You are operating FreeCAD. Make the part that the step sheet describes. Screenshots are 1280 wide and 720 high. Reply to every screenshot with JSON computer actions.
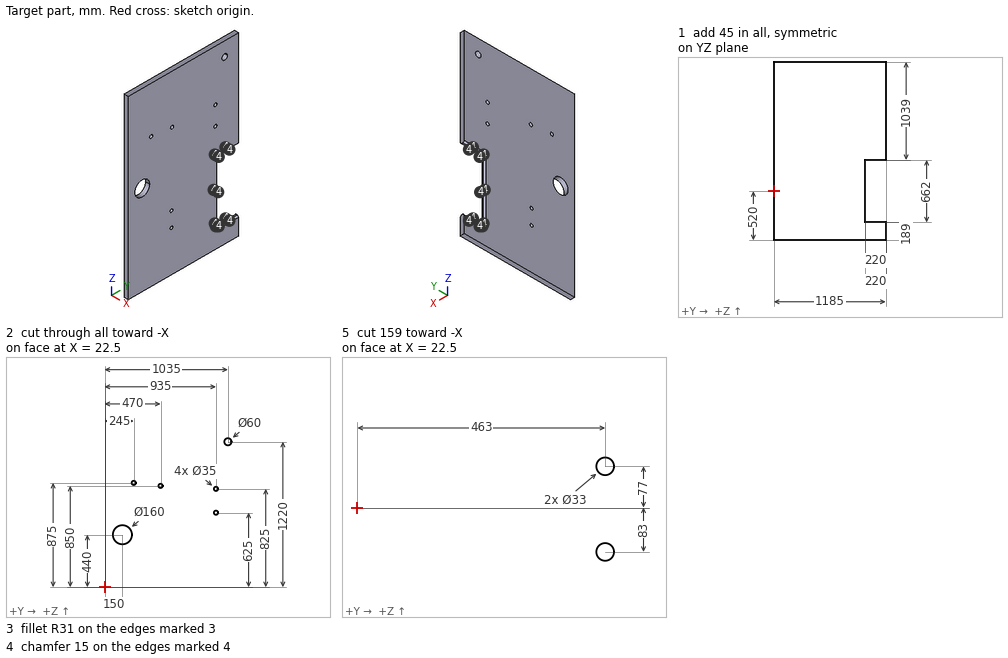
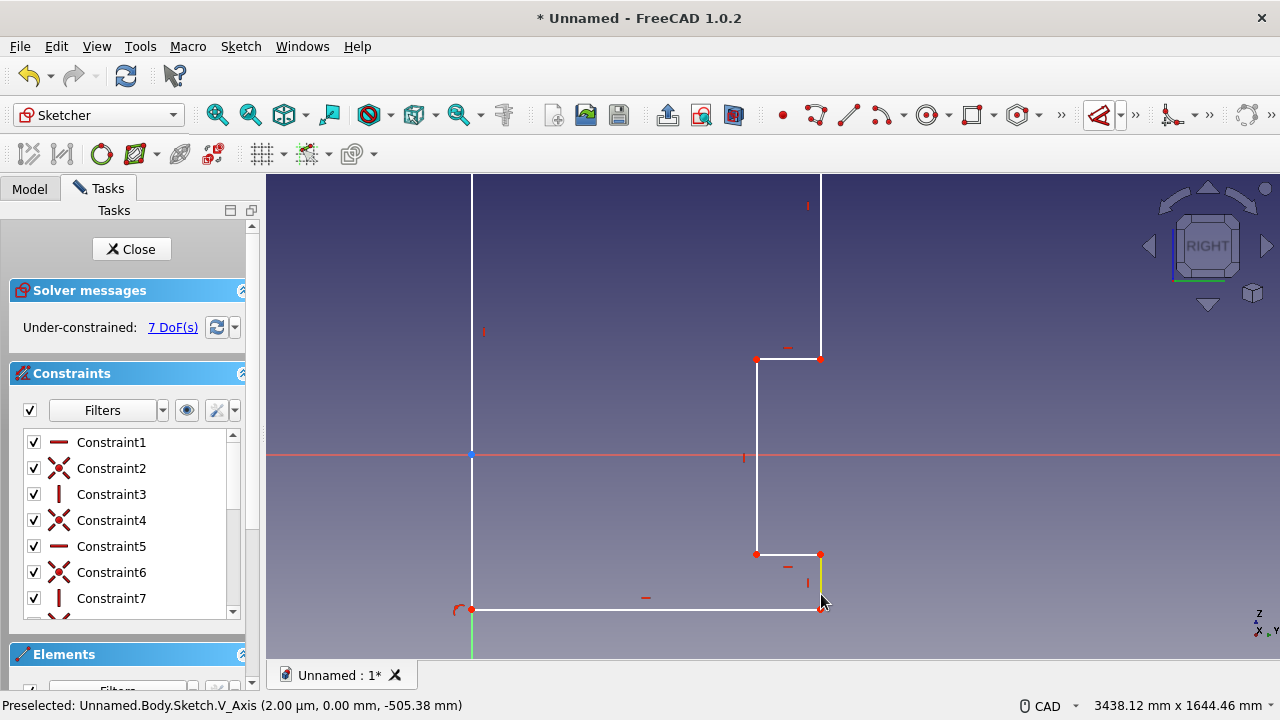
{"action": "left_click", "coordinate": [821, 593]}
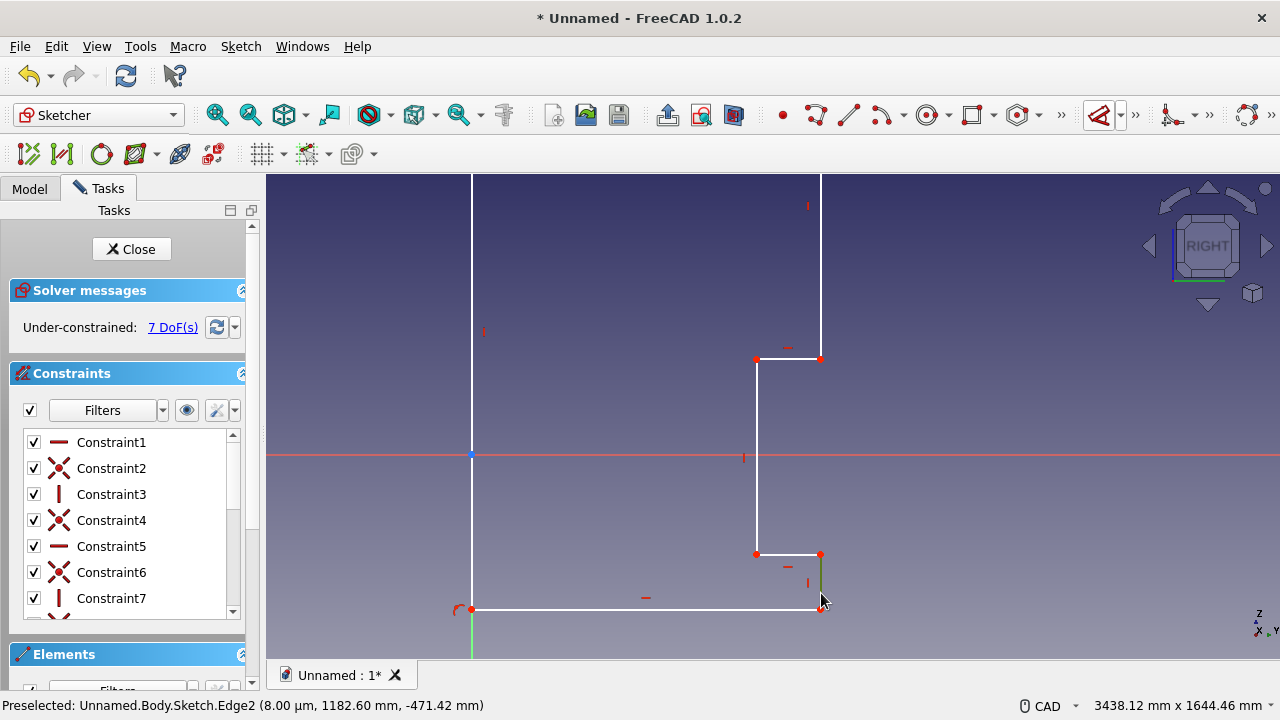
{"action": "left_click", "coordinate": [1120, 116]}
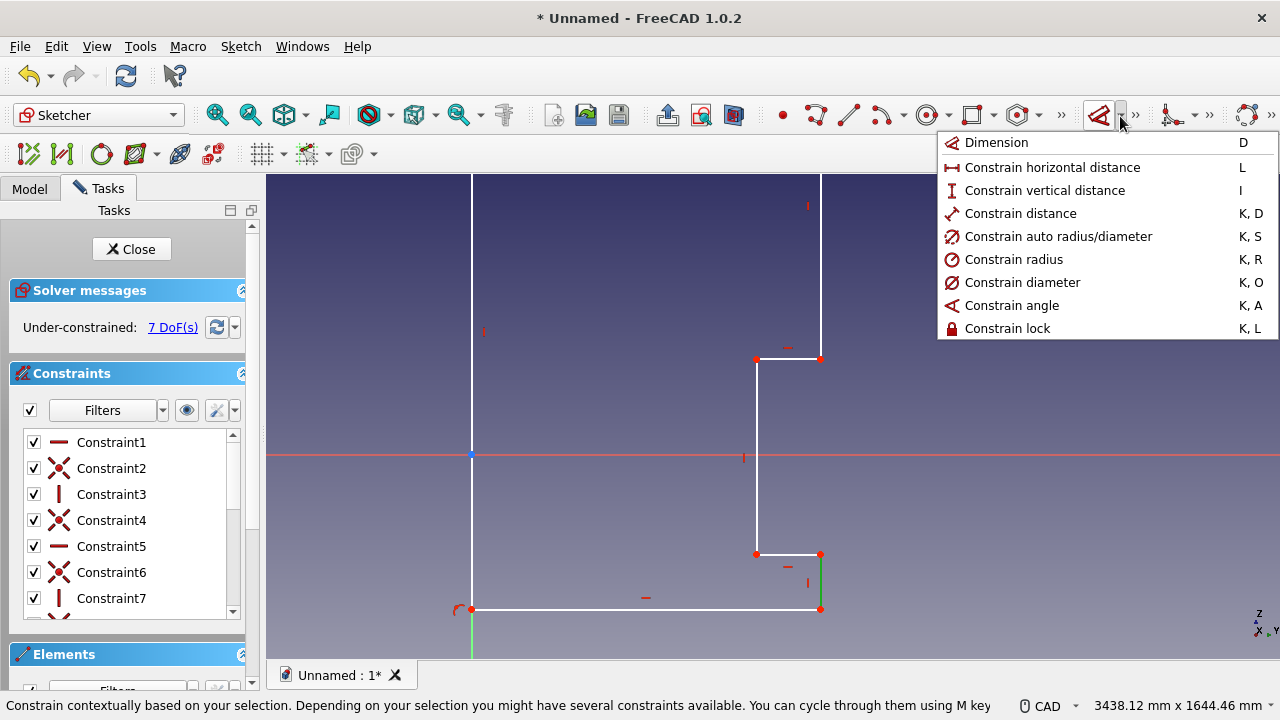
{"action": "left_click", "coordinate": [1108, 190]}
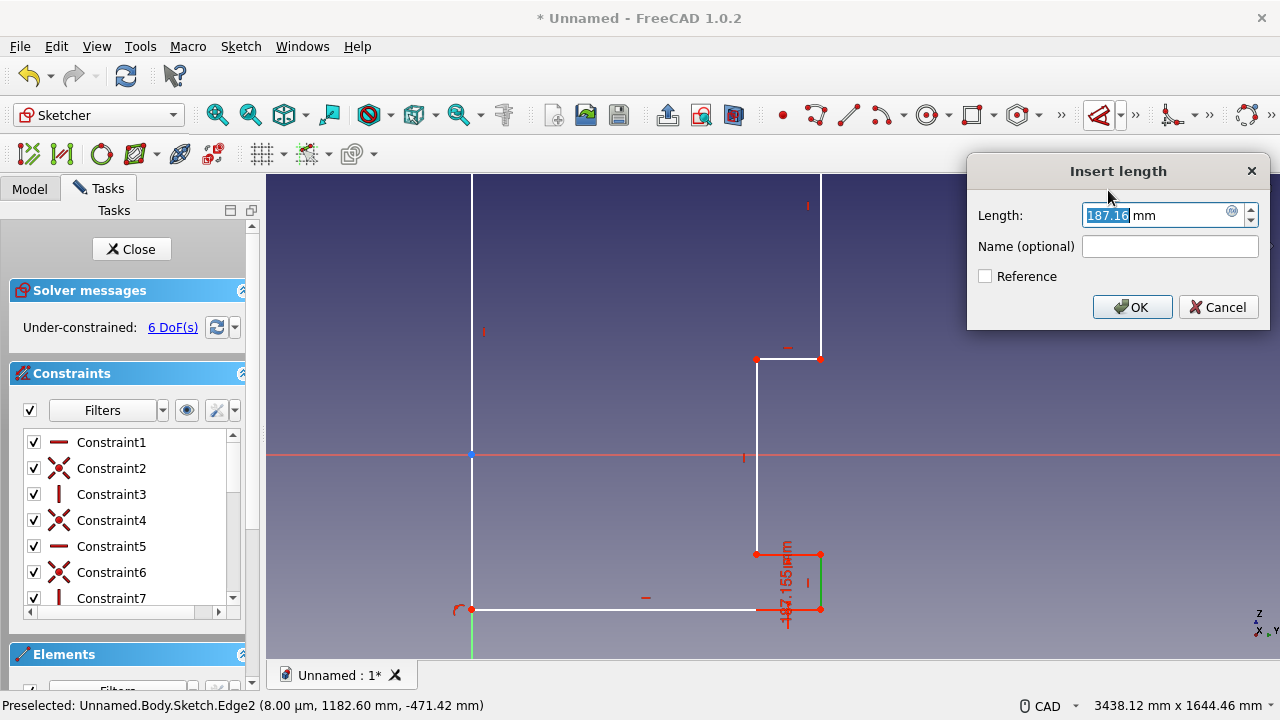
{"action": "type", "text": "189"}
{"action": "key", "text": "Return"}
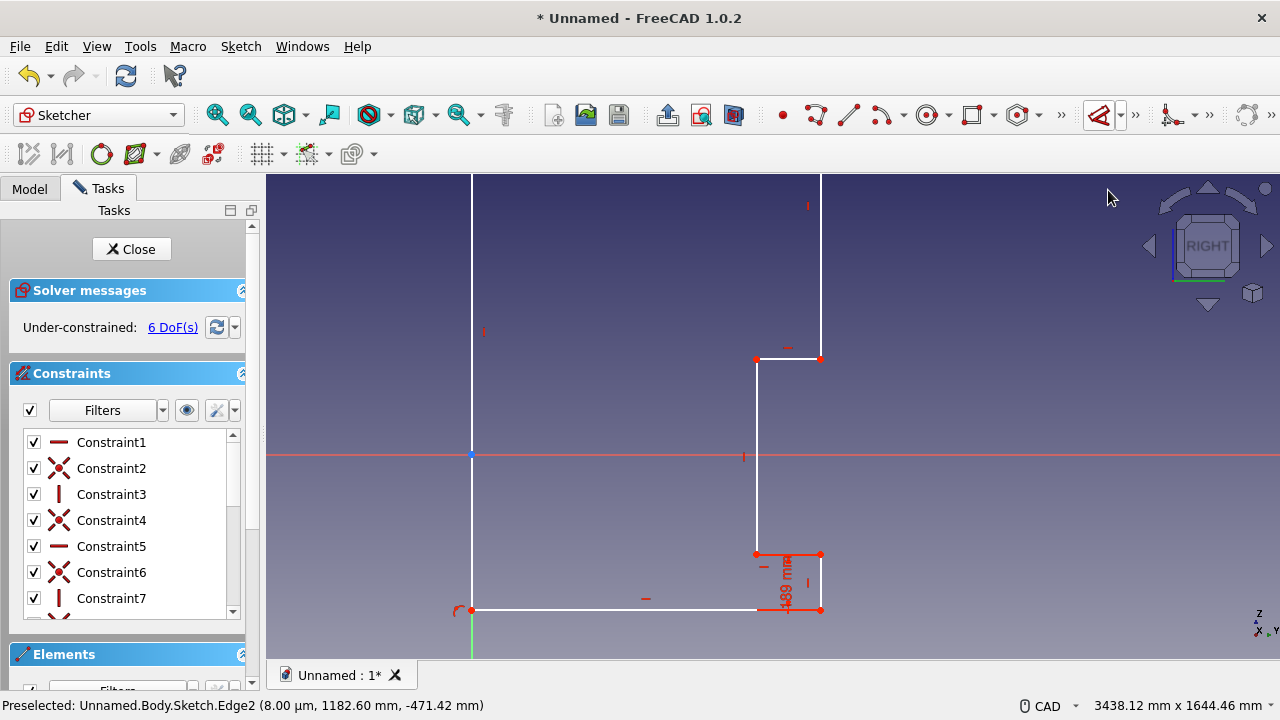
{"action": "left_click", "coordinate": [801, 555]}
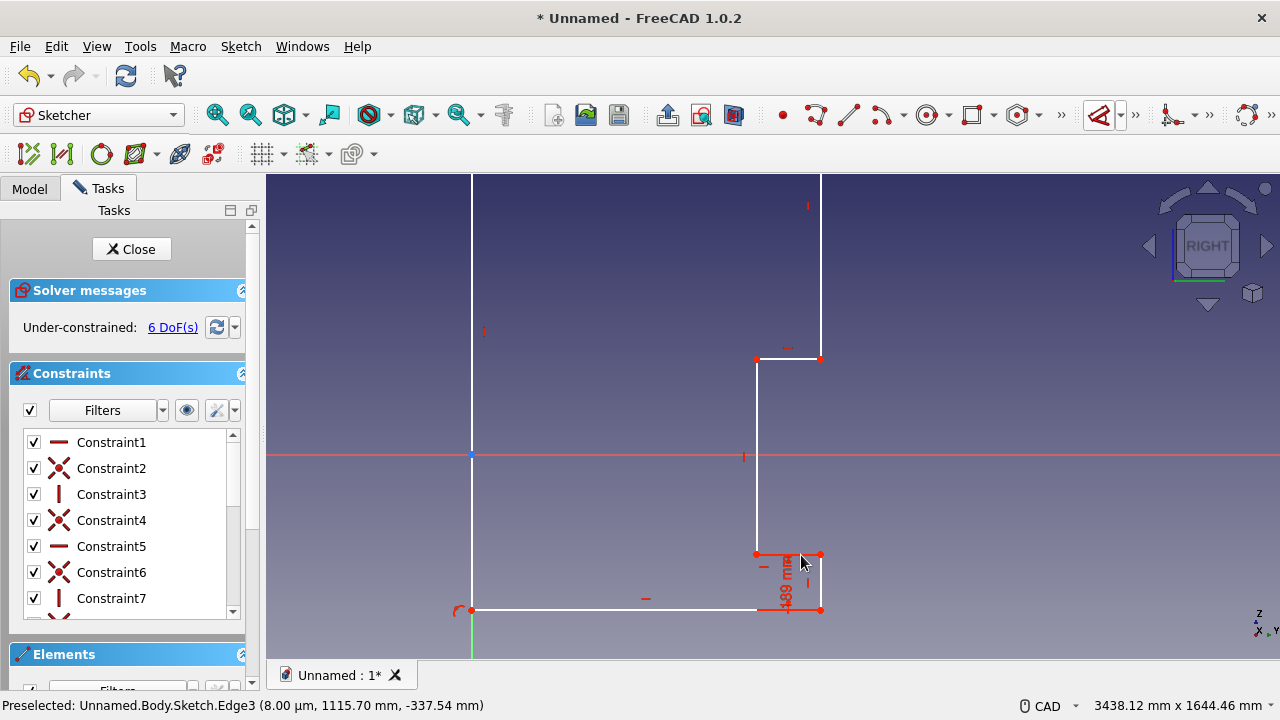
{"action": "left_click", "coordinate": [1120, 116]}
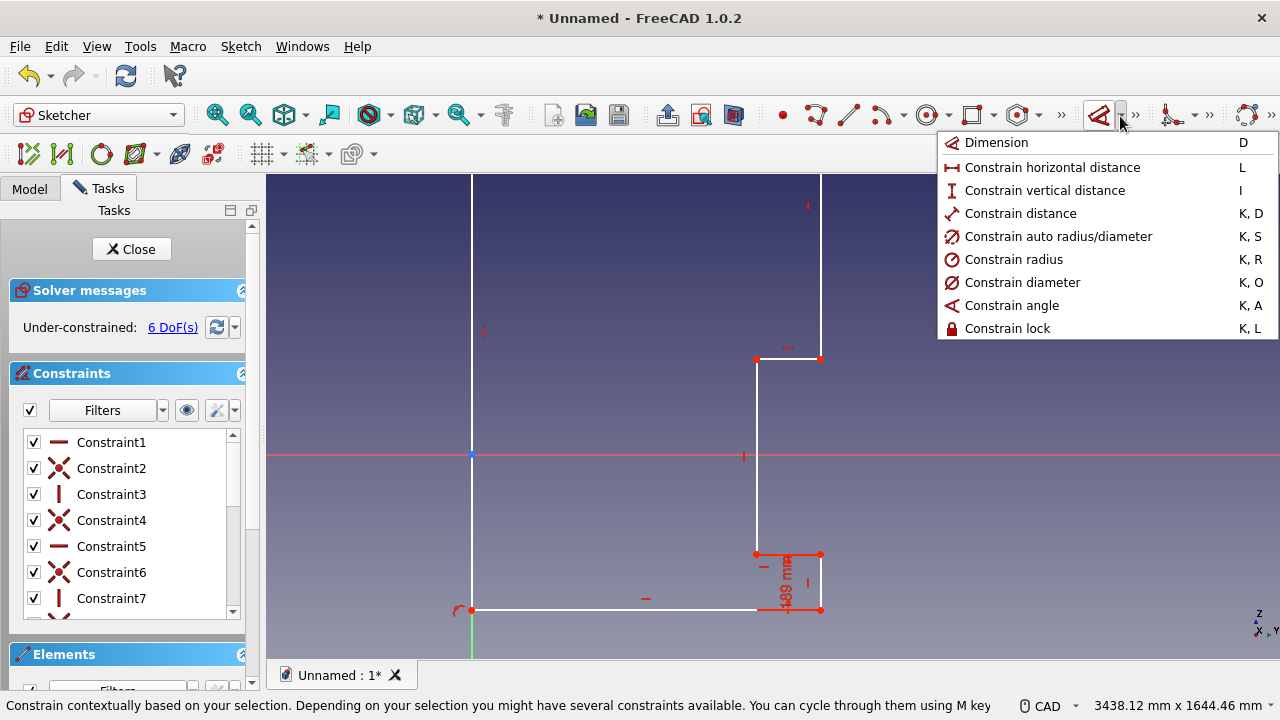
{"action": "left_click", "coordinate": [1108, 168]}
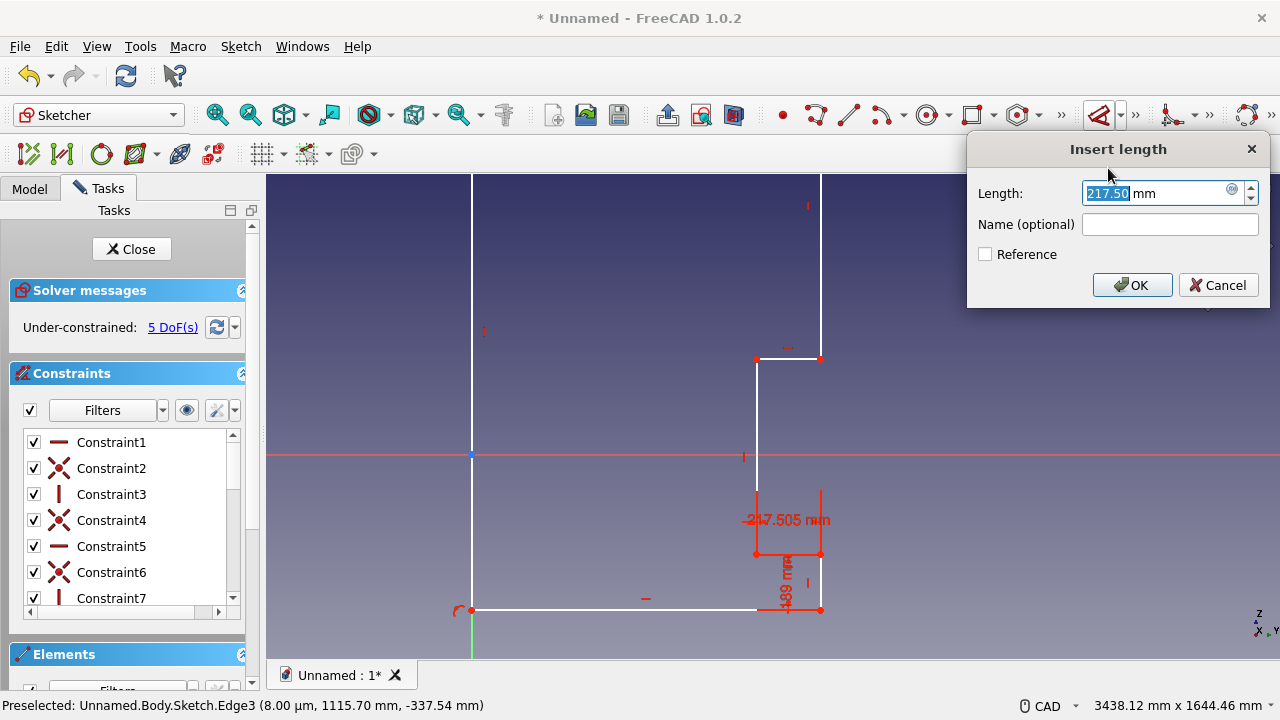
{"action": "type", "text": "220"}
{"action": "key", "text": "Return"}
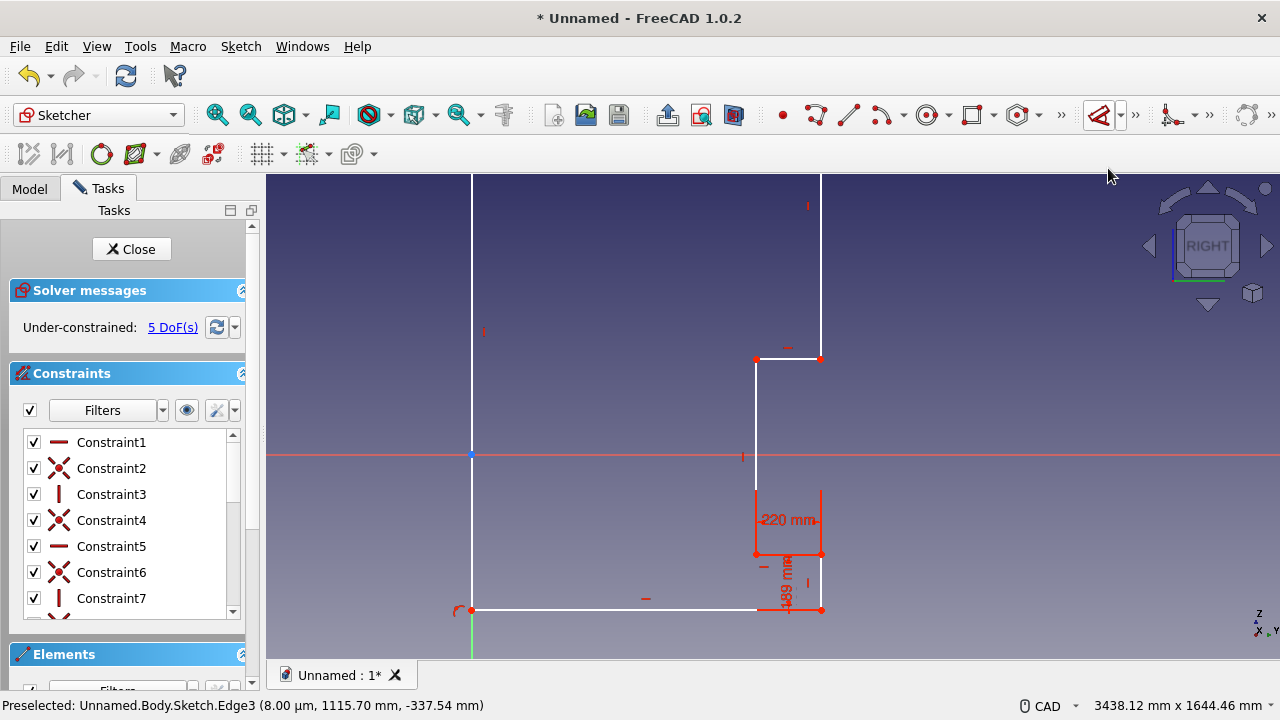
{"action": "left_click", "coordinate": [756, 496]}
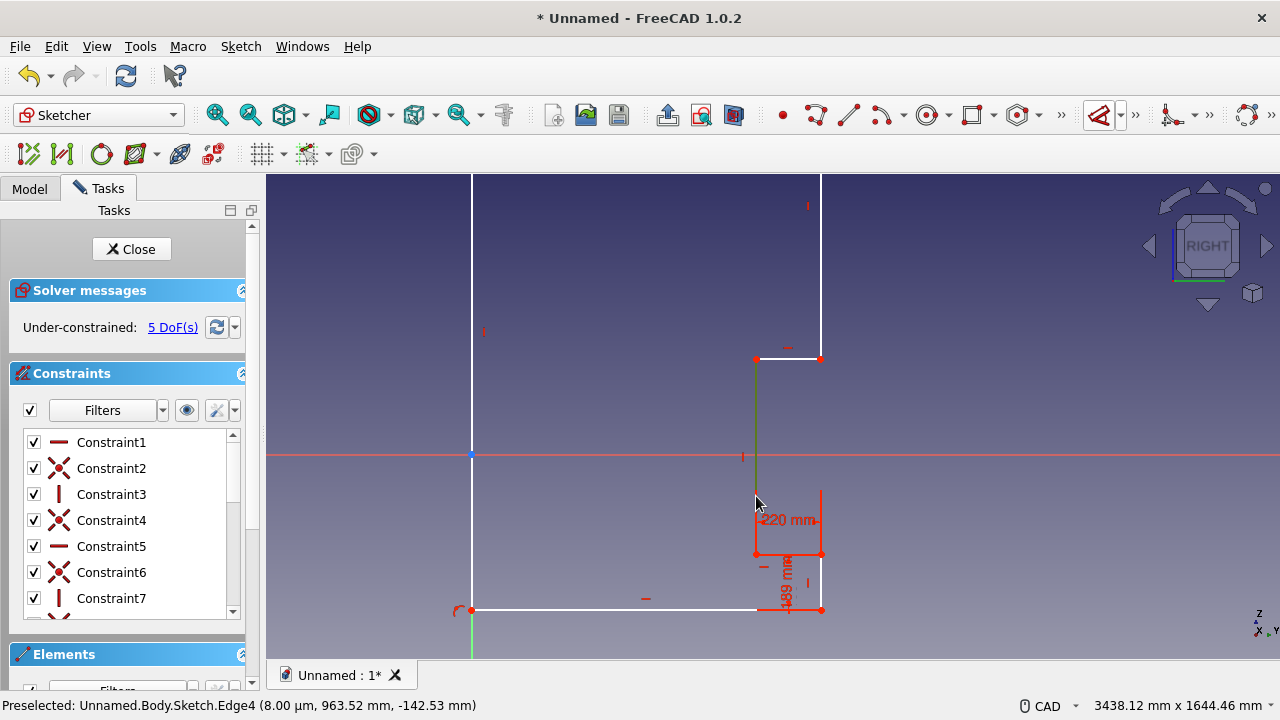
{"action": "left_click", "coordinate": [1120, 116]}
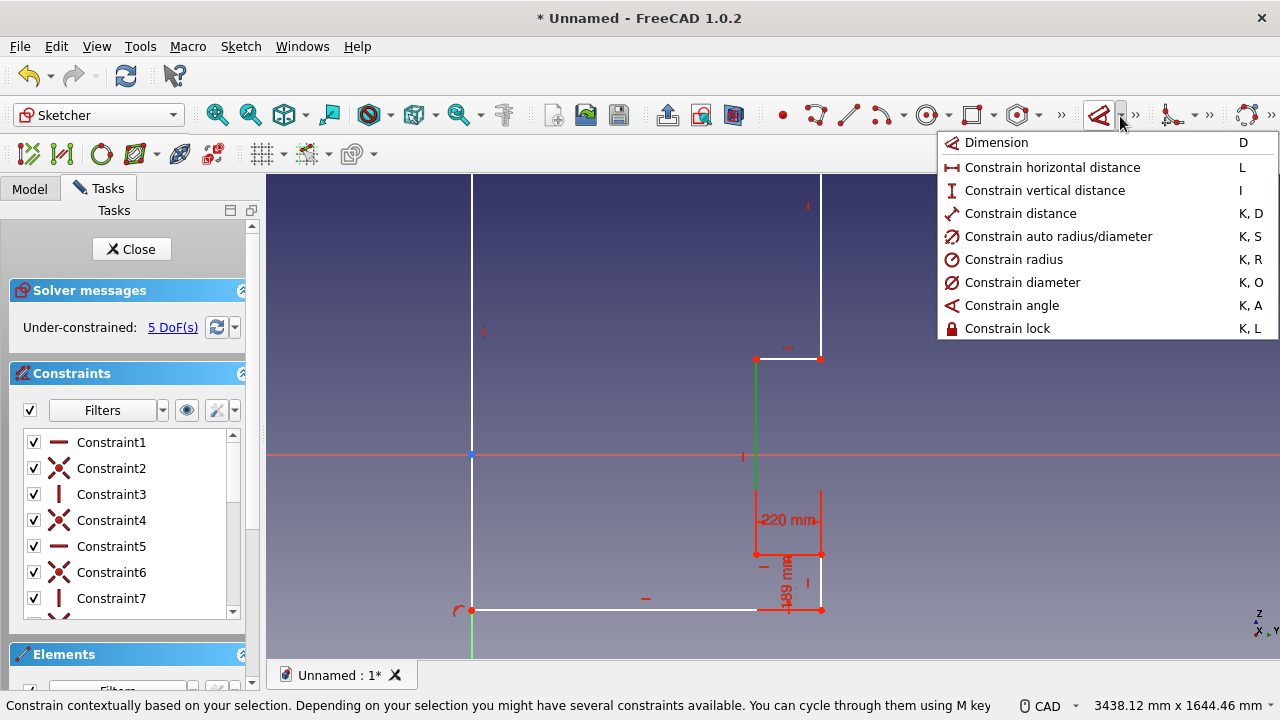
{"action": "left_click", "coordinate": [1108, 190]}